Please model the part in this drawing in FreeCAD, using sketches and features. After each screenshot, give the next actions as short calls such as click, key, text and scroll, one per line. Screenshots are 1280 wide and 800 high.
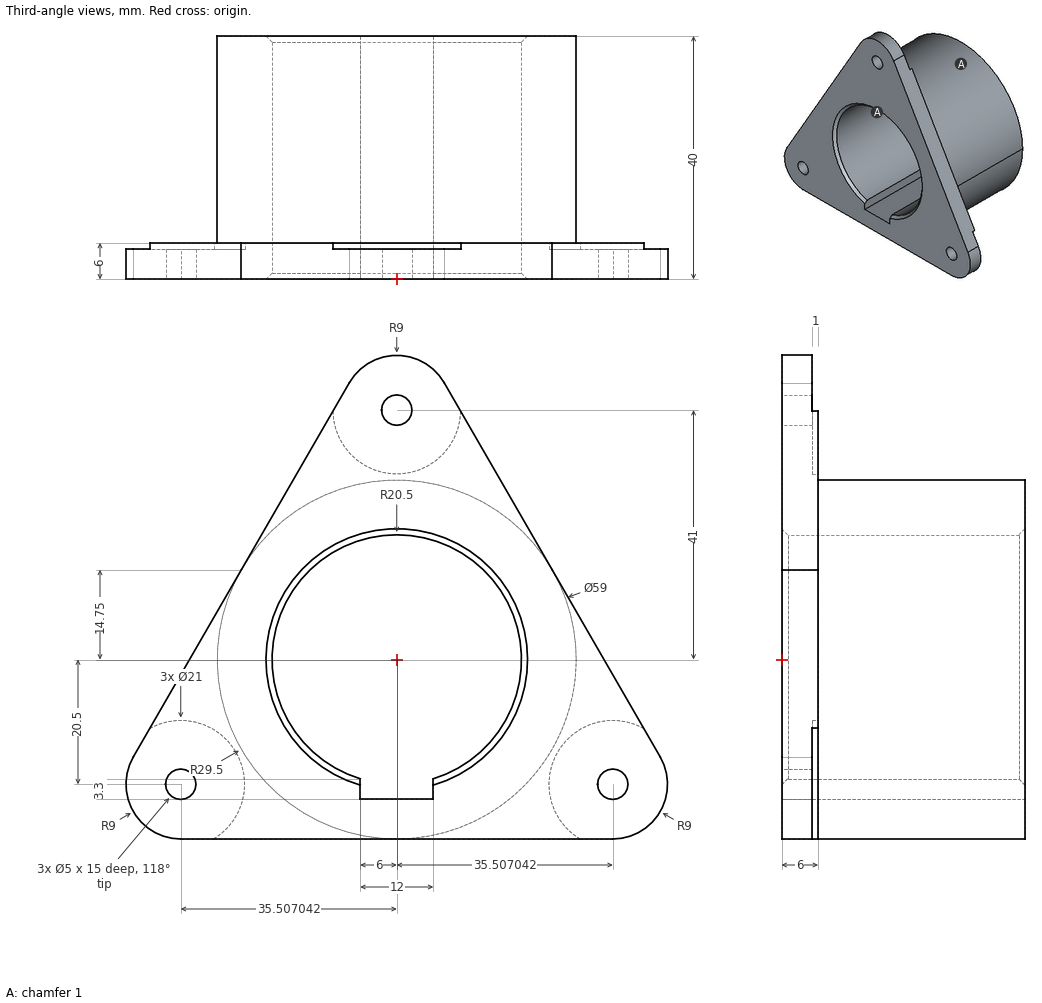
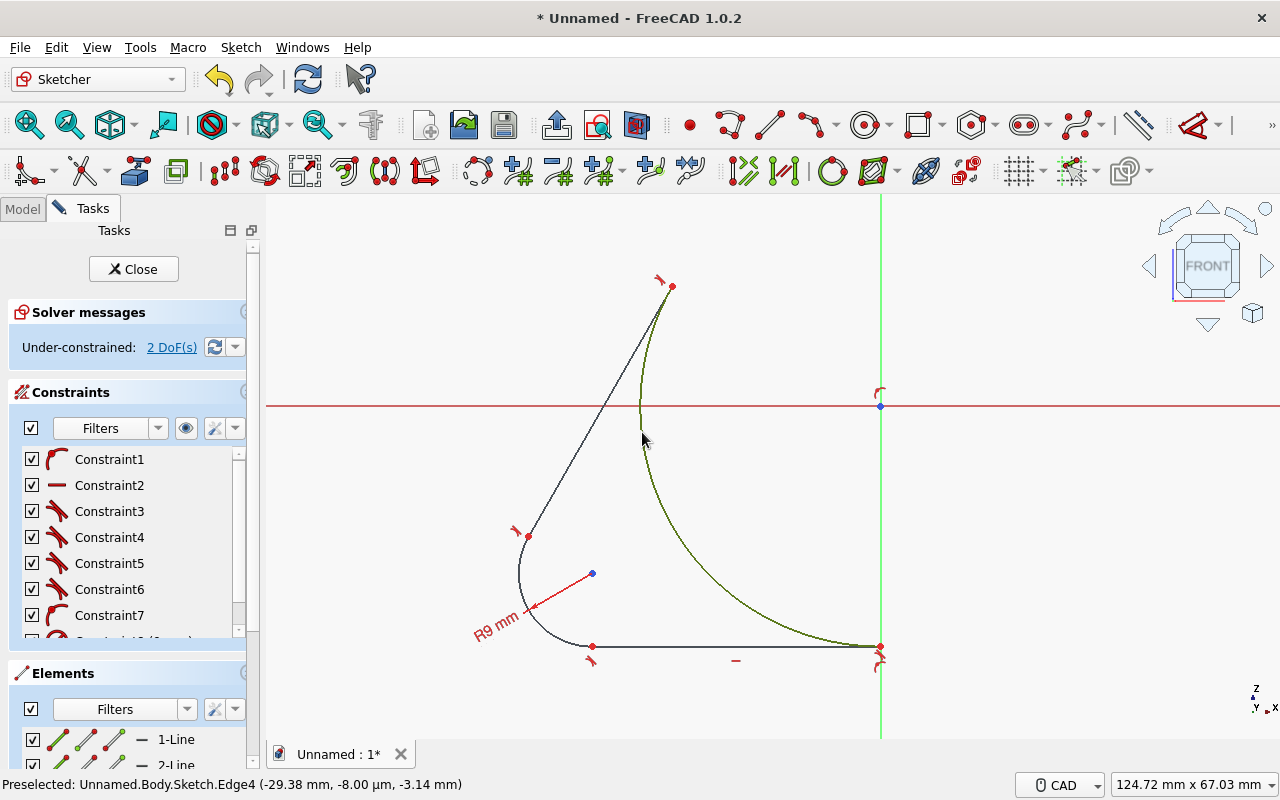
key(k)
key(r)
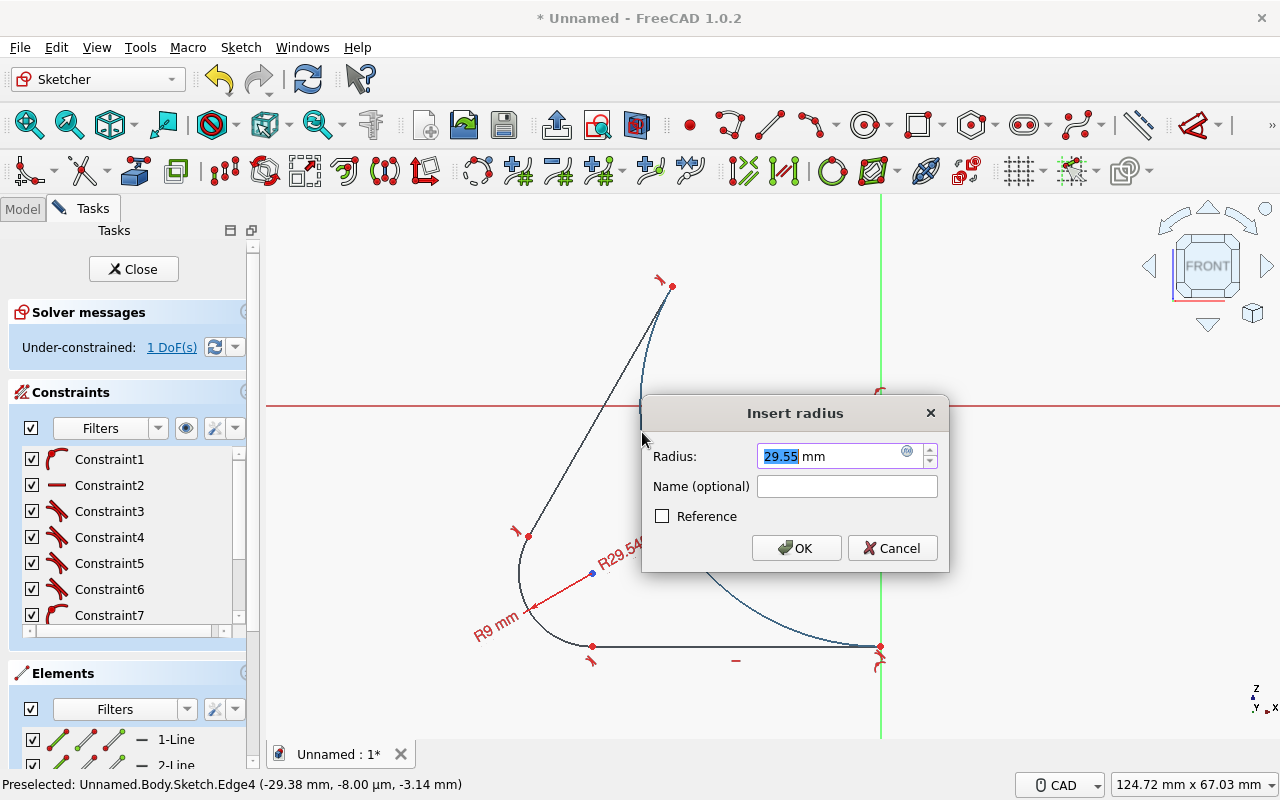
text(29.5)
key(Return)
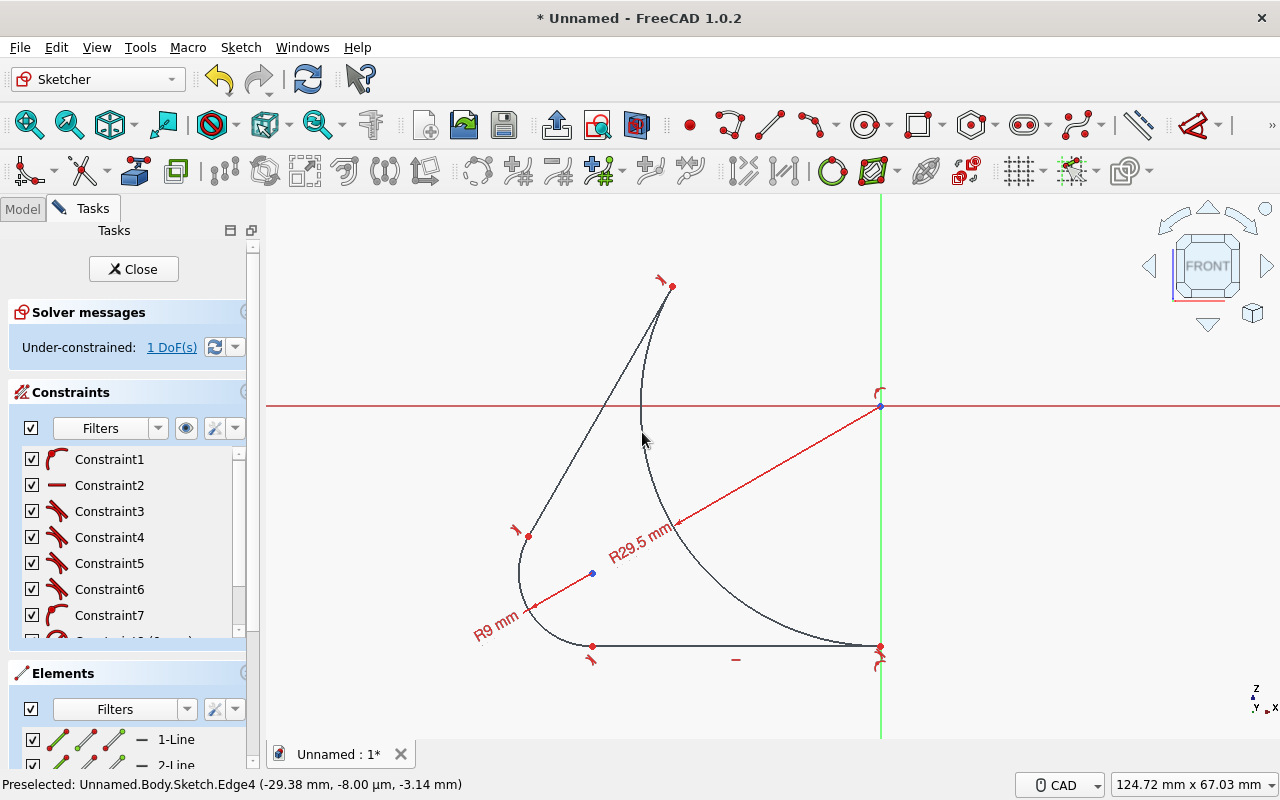
click(673, 287)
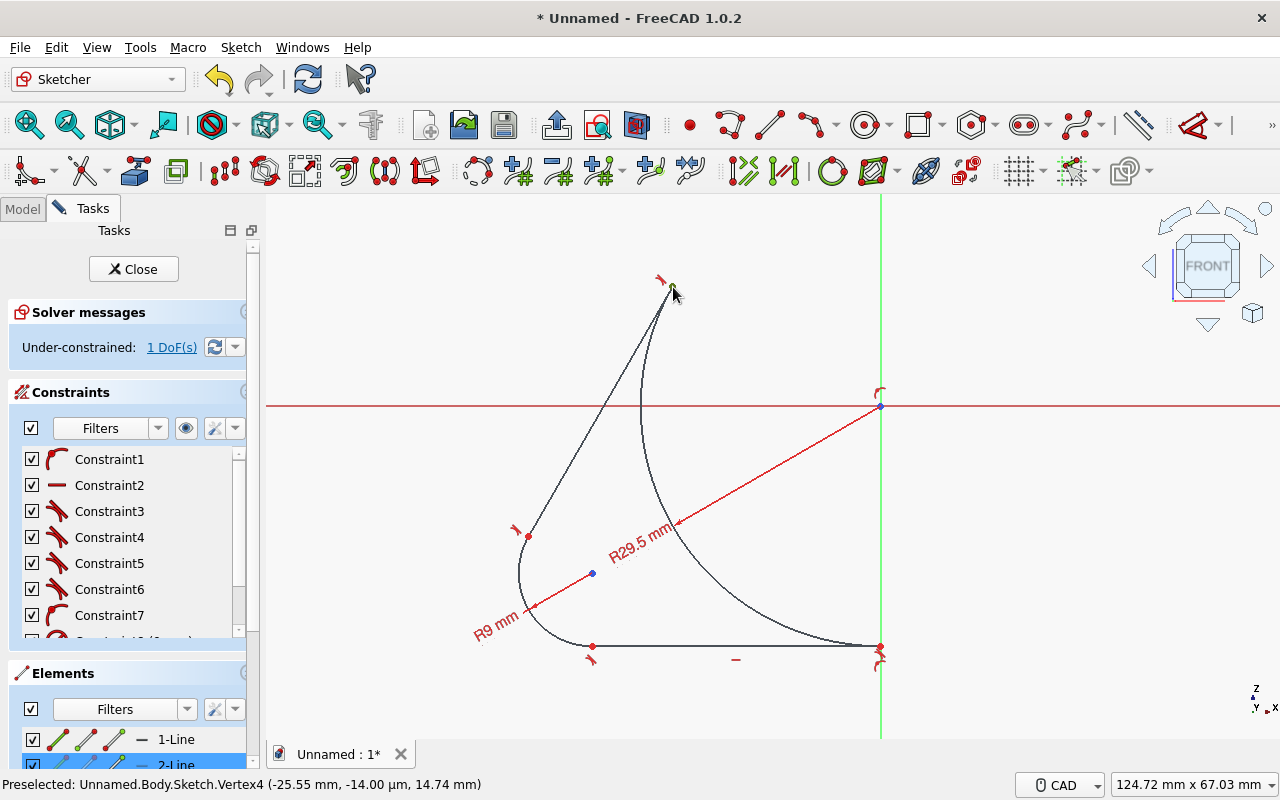
click(1220, 126)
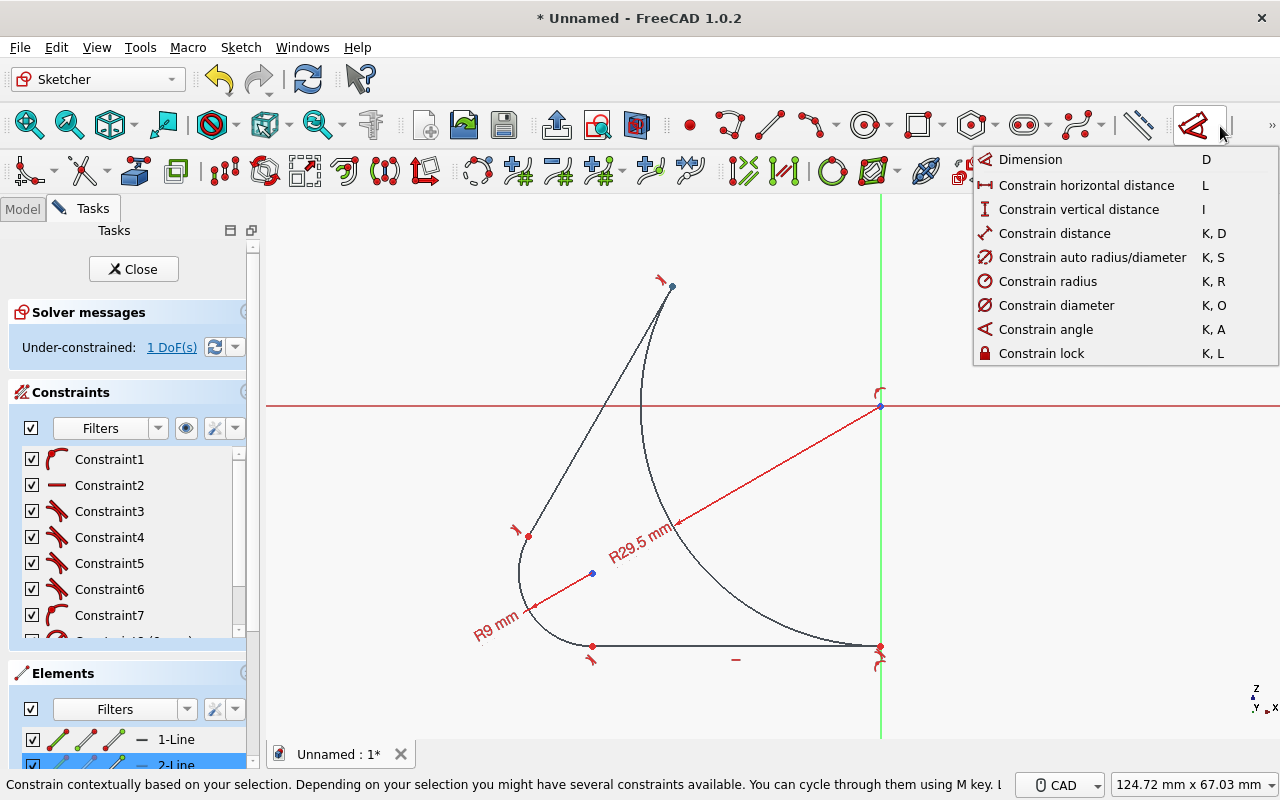
click(1126, 209)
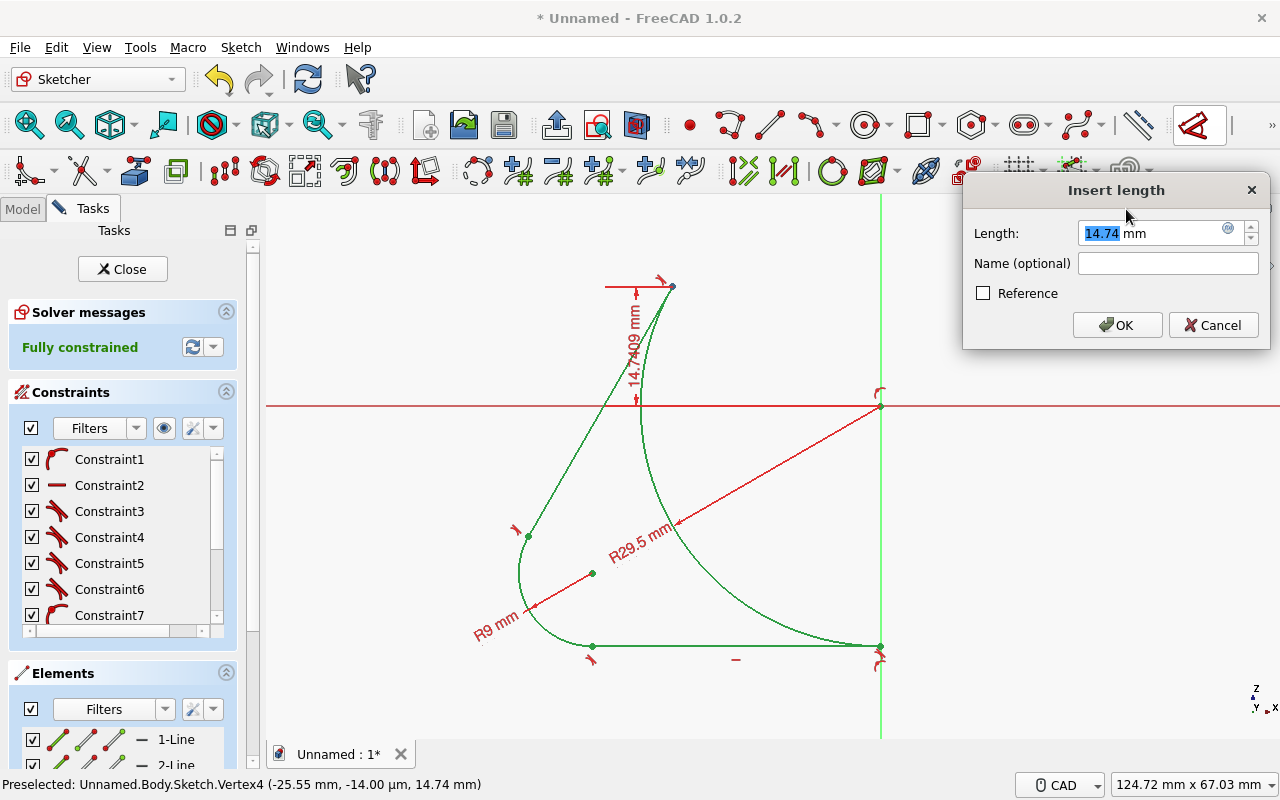
text(14.75)
key(Return)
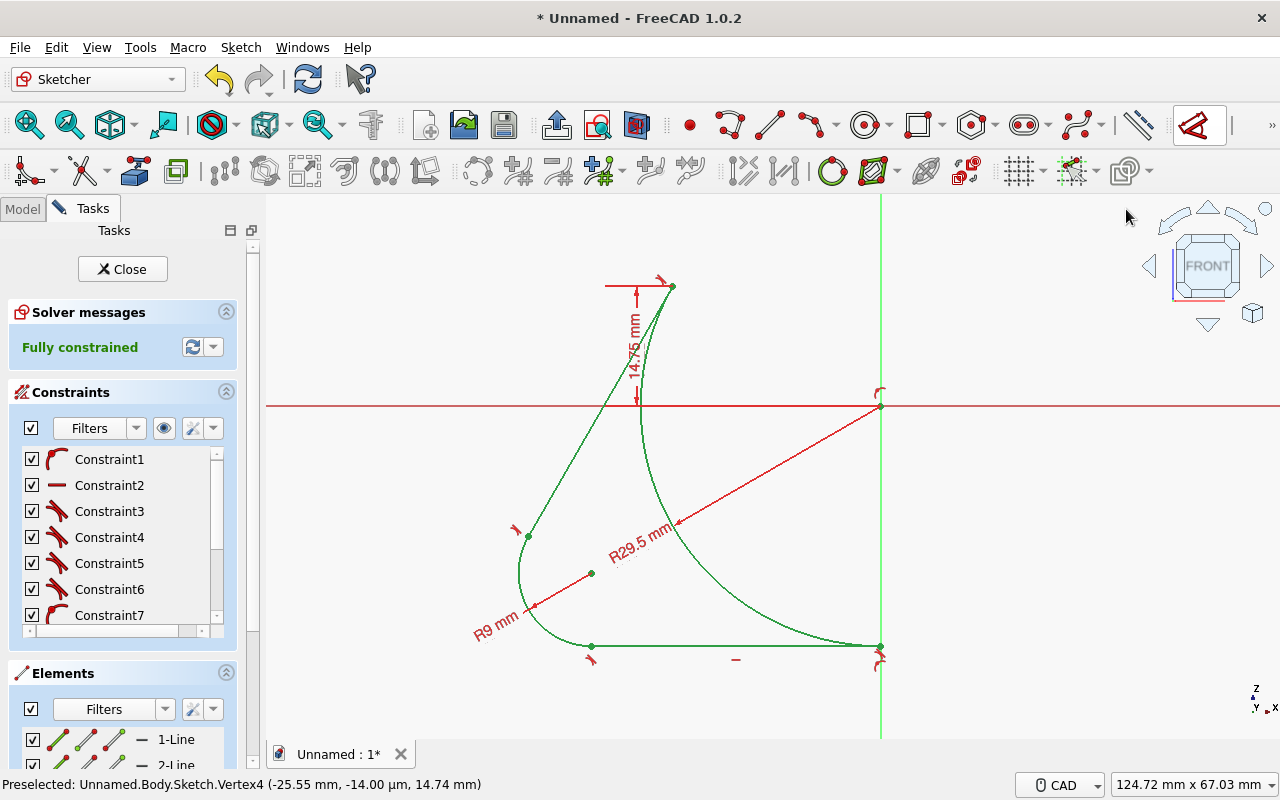
click(123, 269)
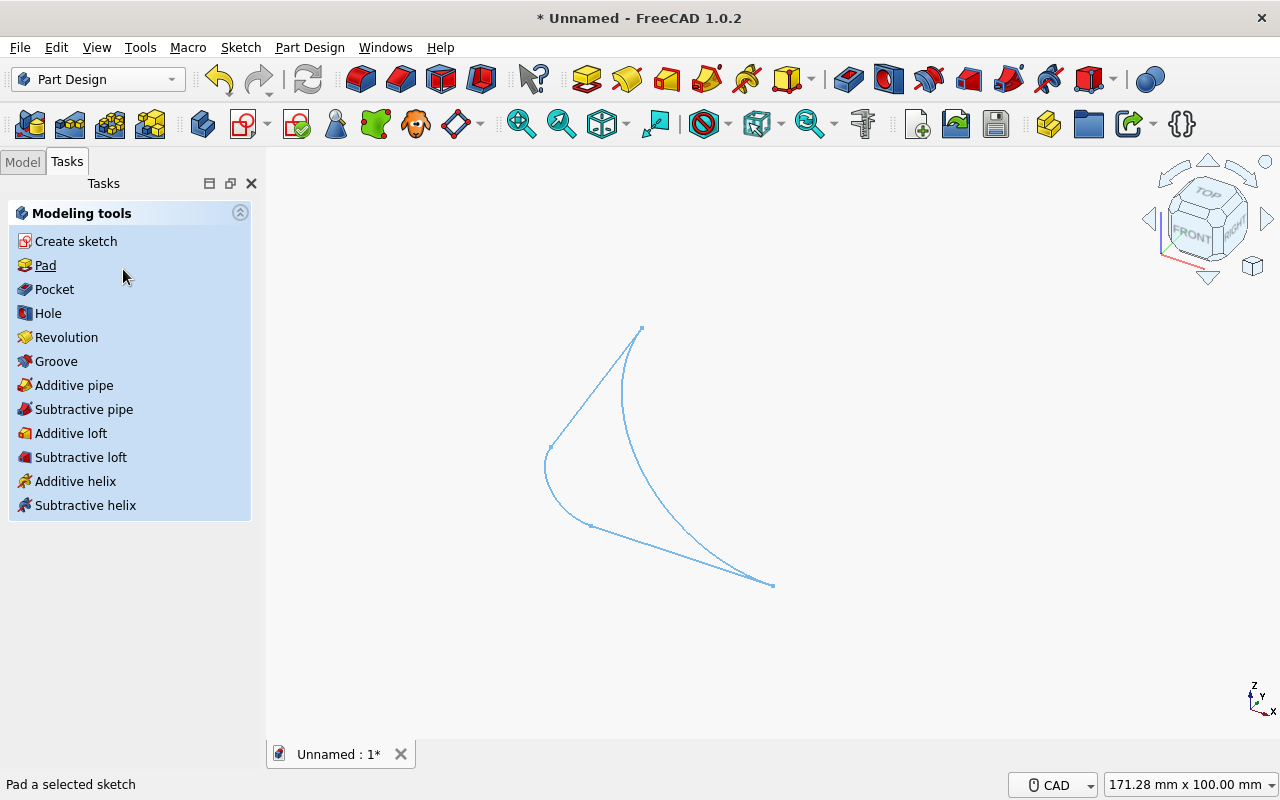
click(588, 80)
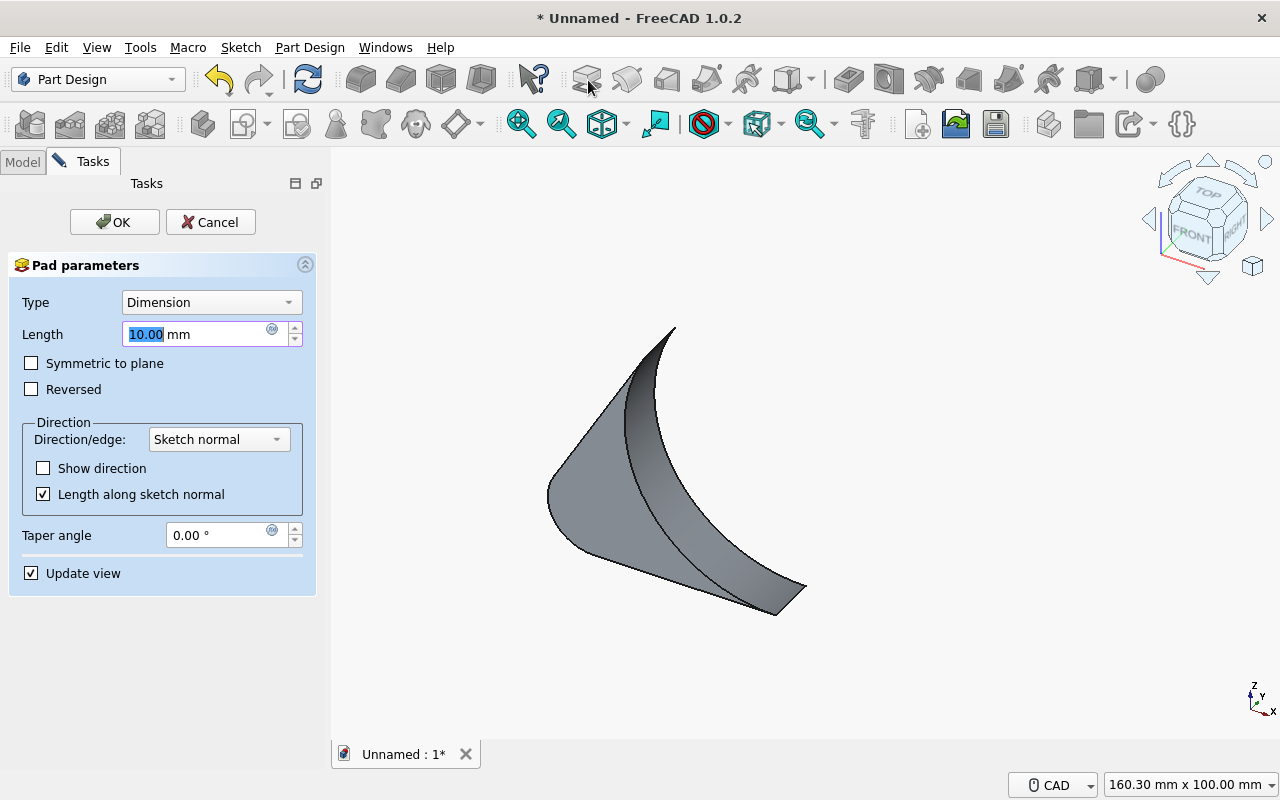
text(6)
key(Tab)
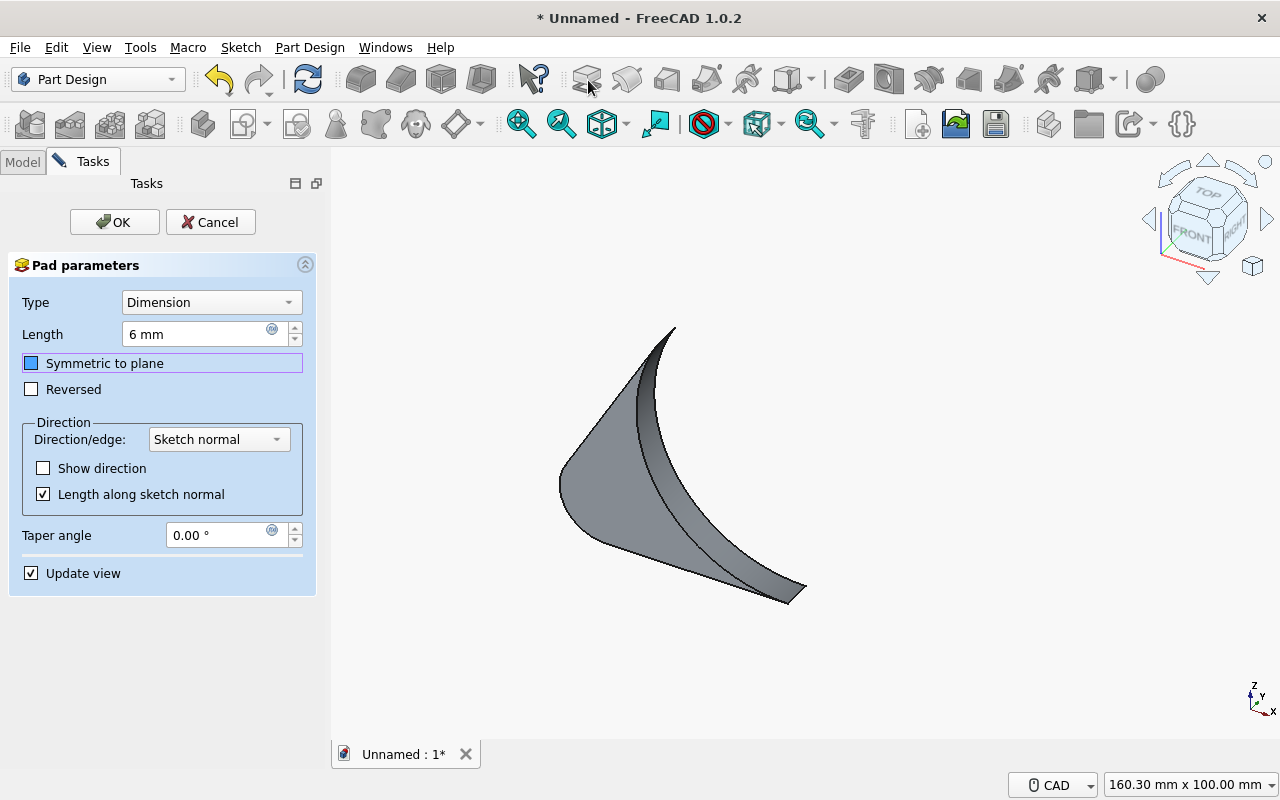
click(30, 389)